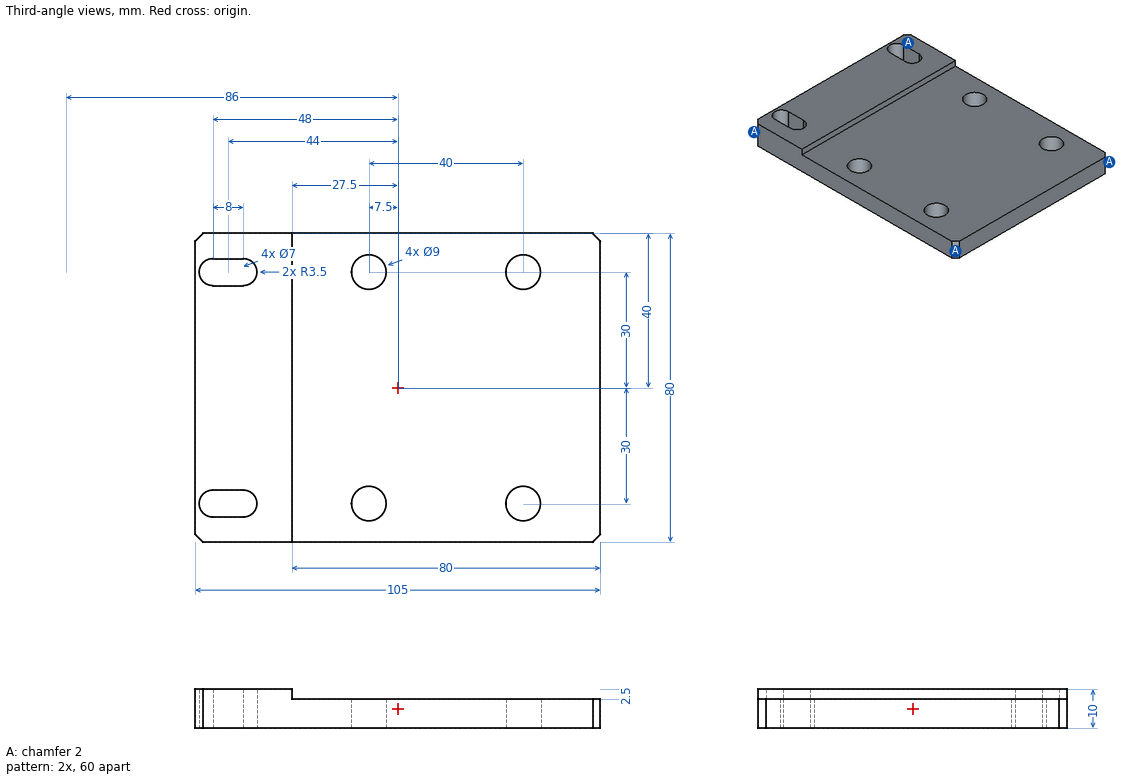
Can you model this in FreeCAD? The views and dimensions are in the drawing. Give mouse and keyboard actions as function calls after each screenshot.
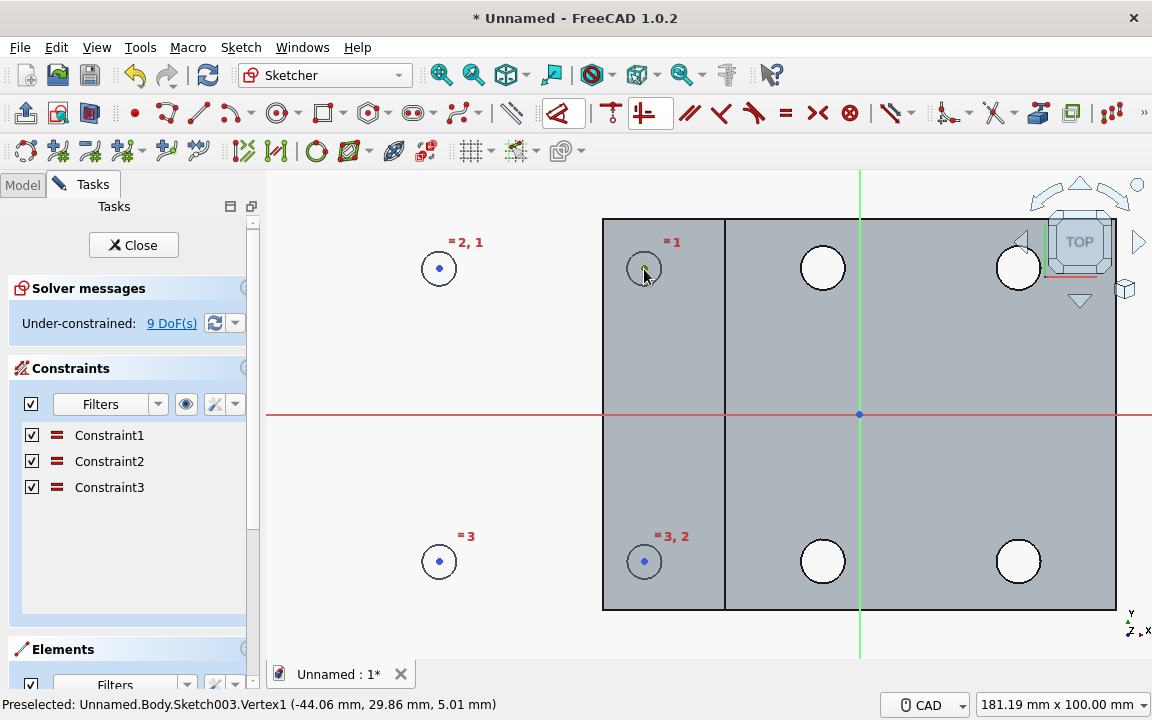
click(439, 269)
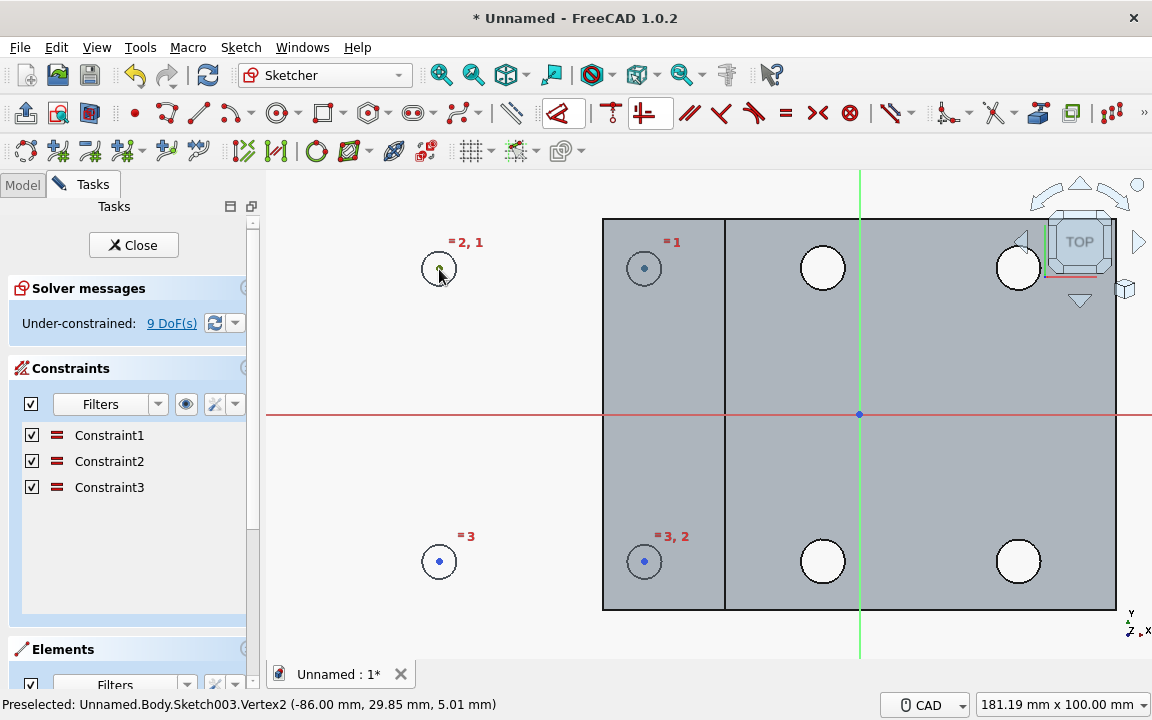
key(h)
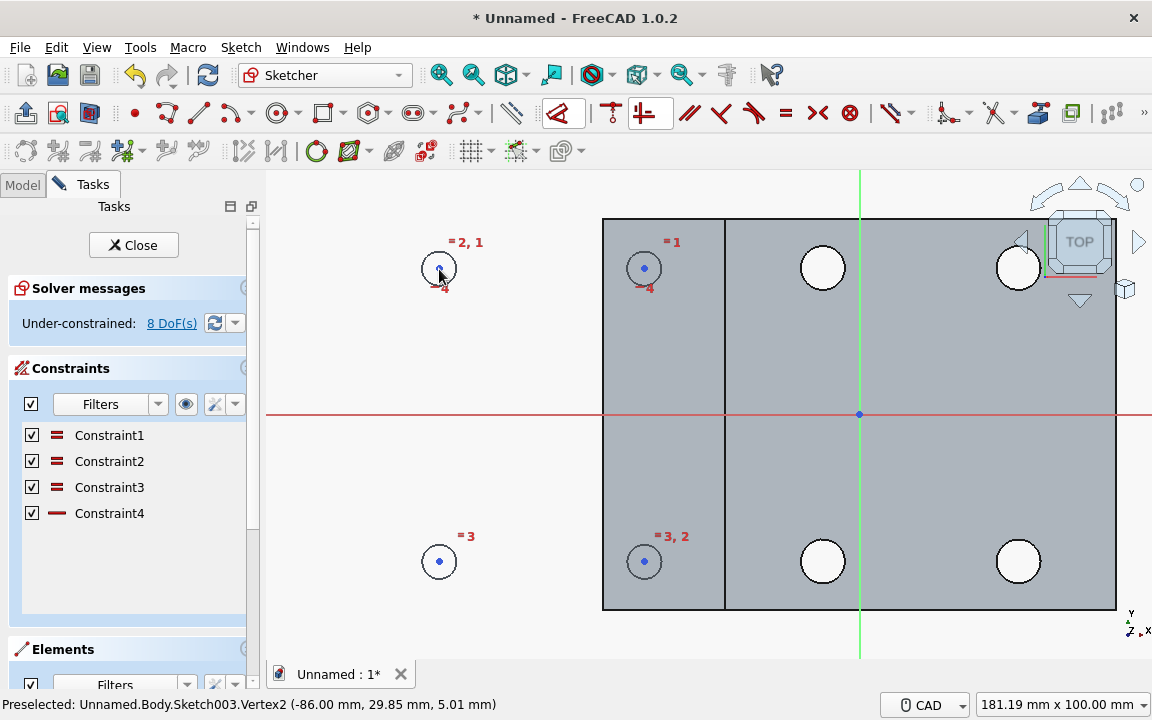
click(644, 269)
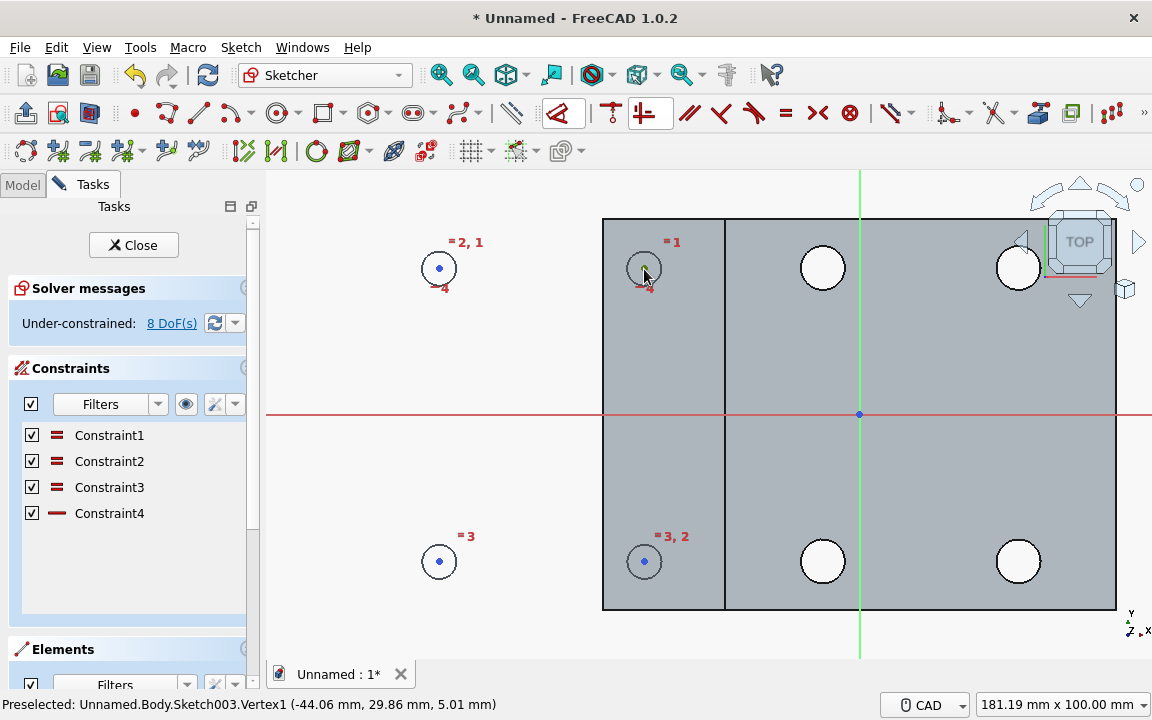
click(644, 562)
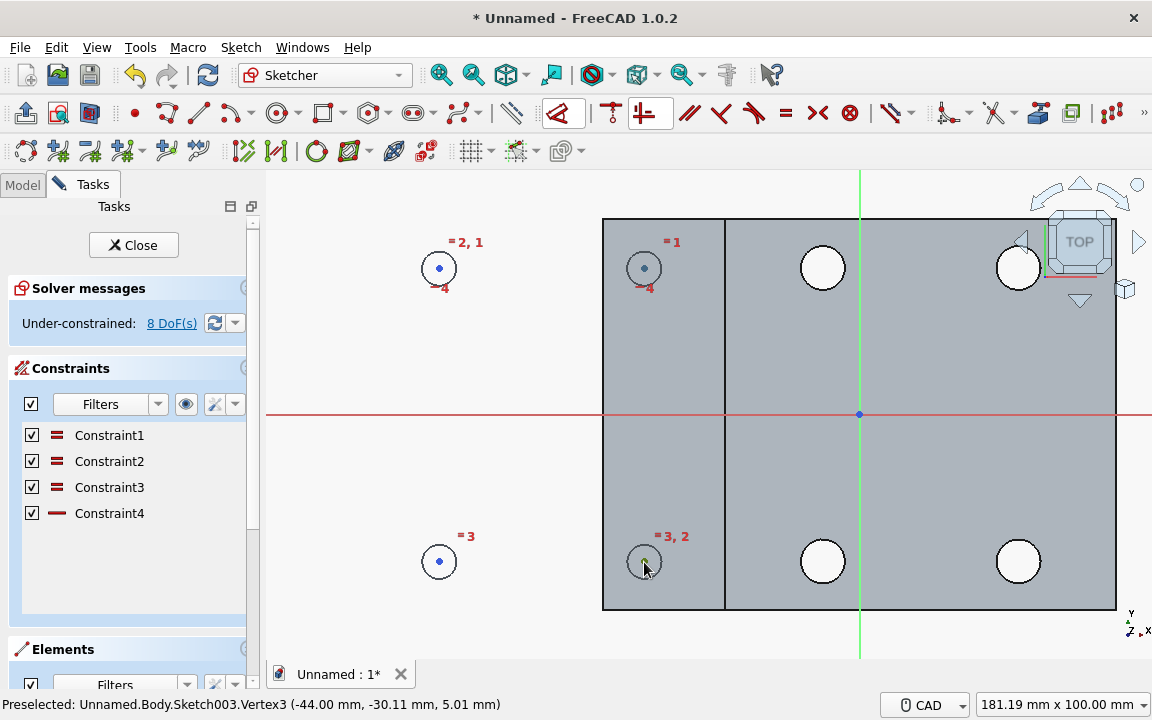
key(v)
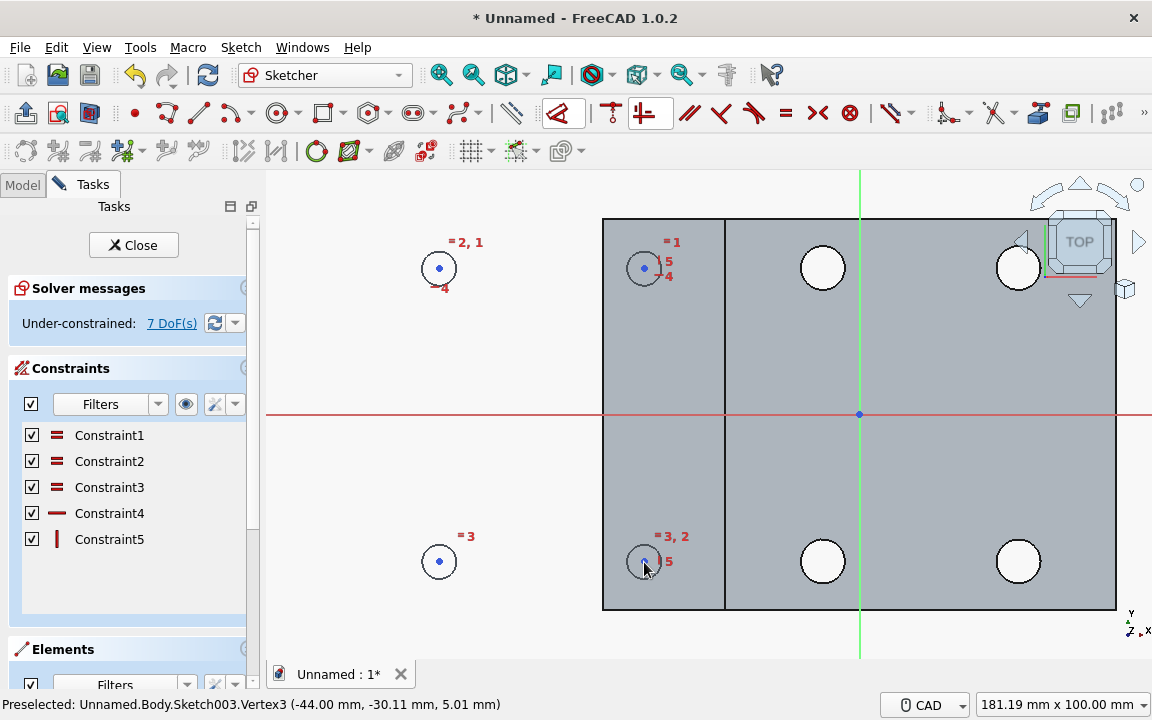
click(439, 269)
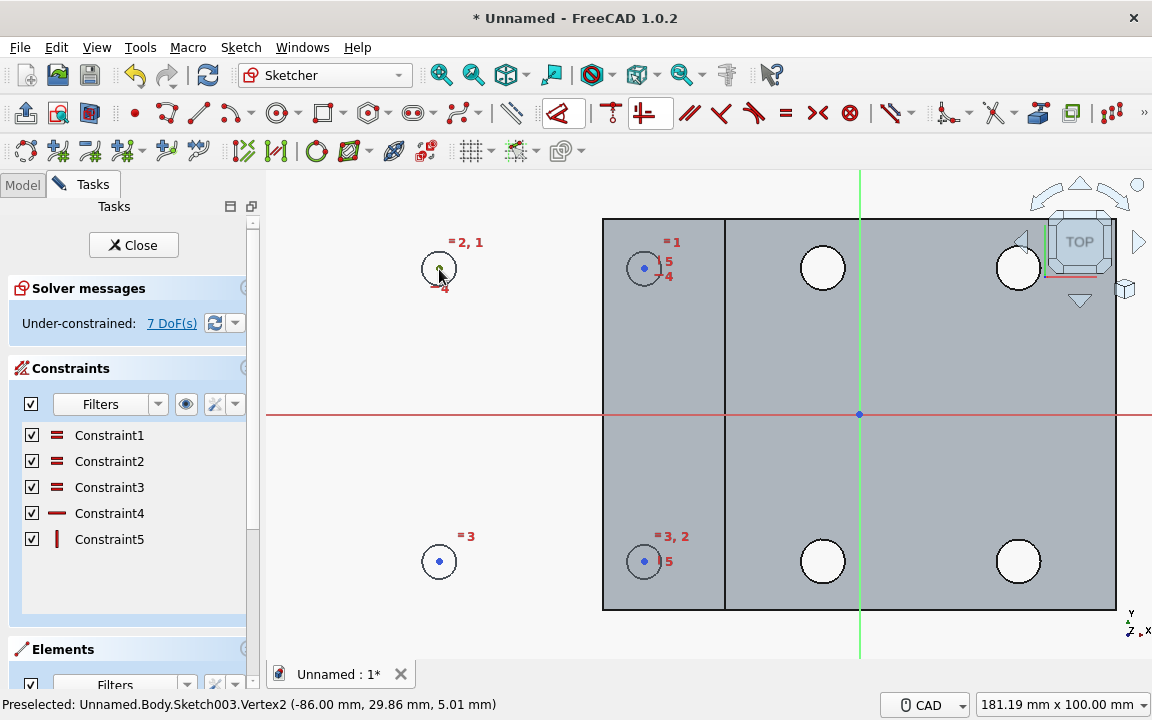
click(439, 562)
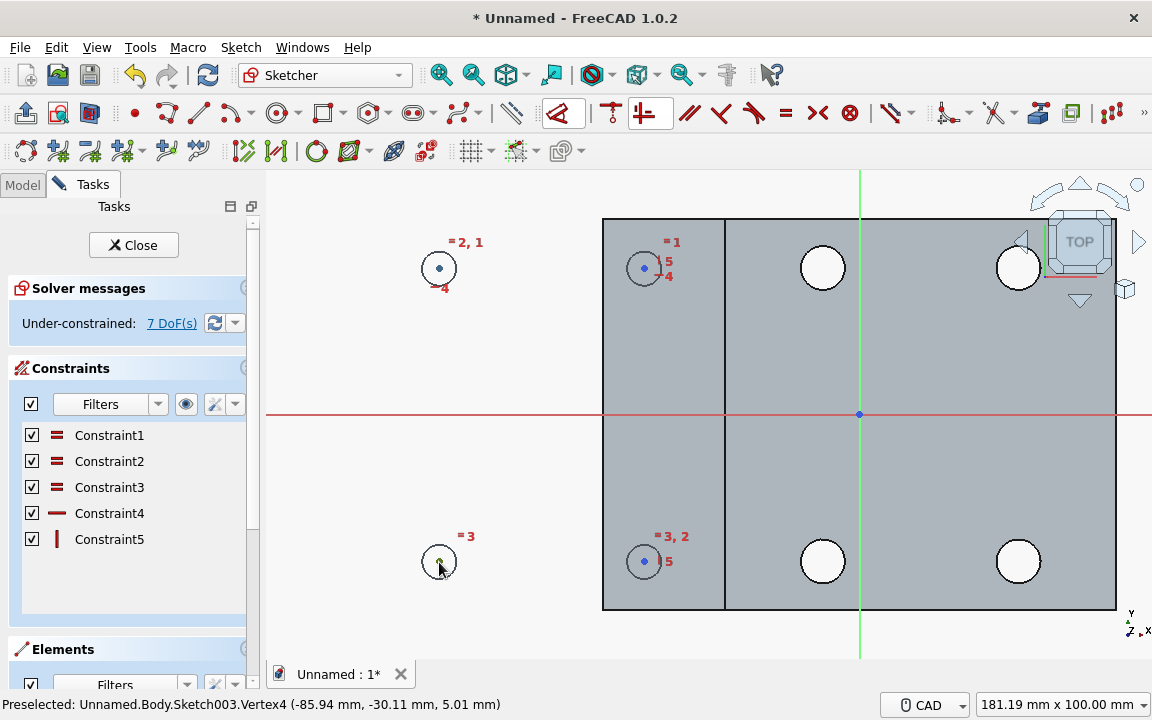
click(668, 114)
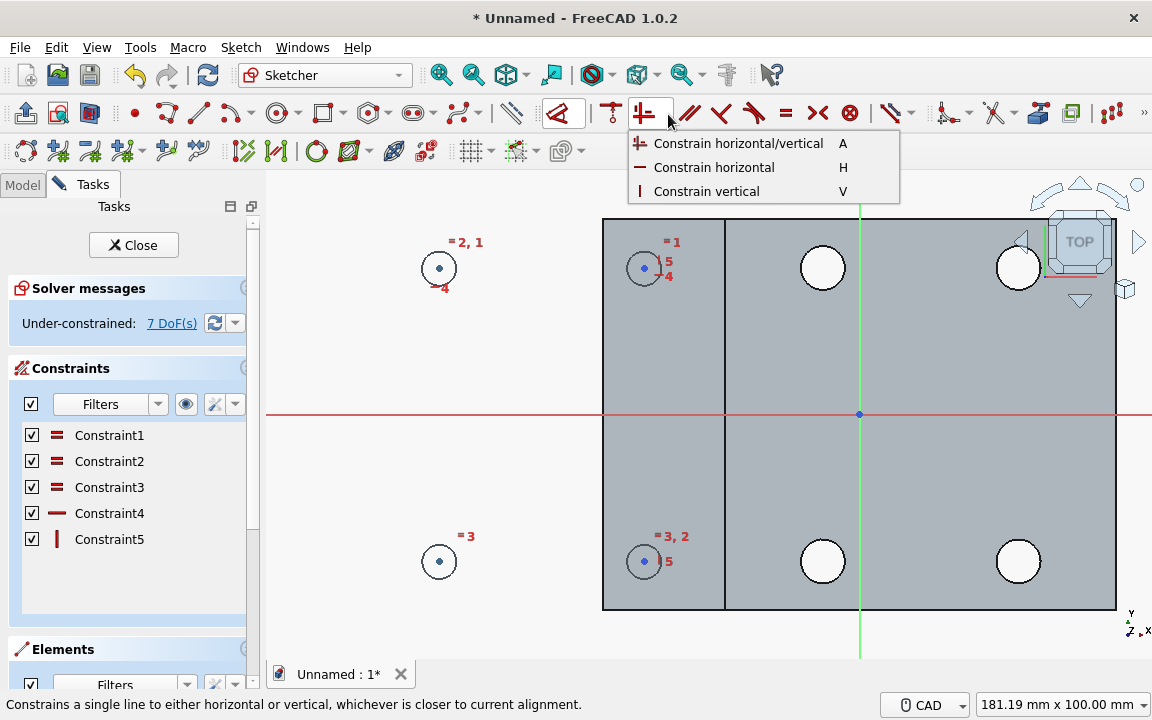
click(764, 191)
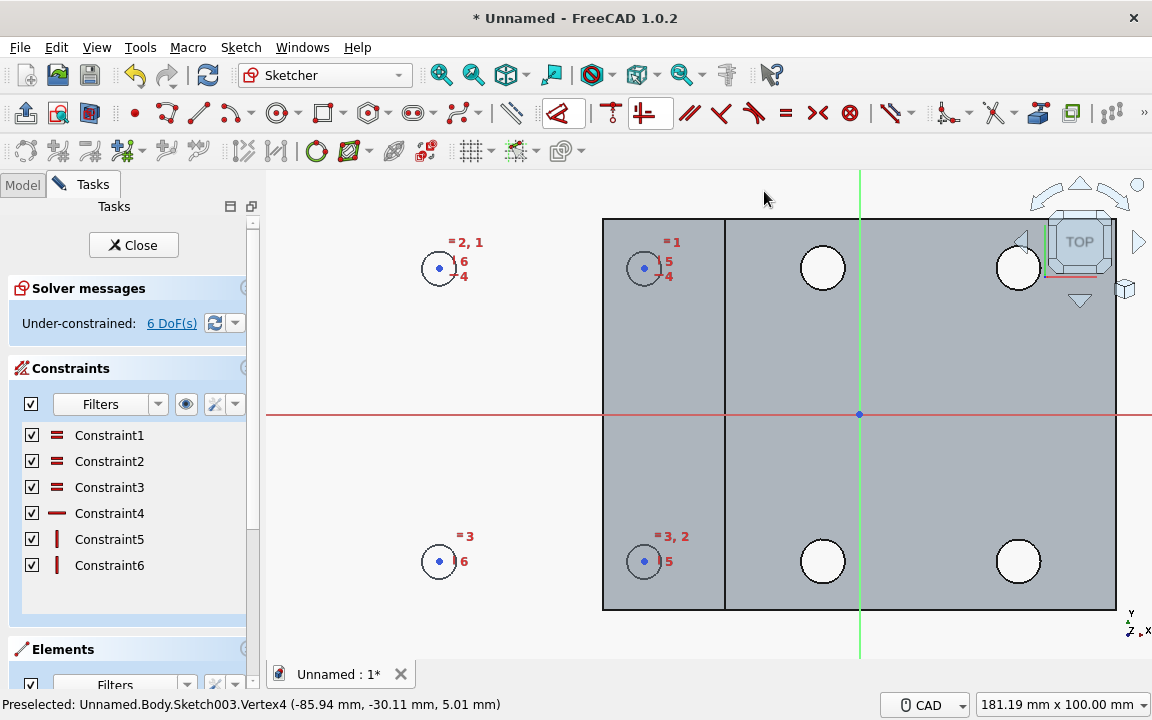
click(644, 562)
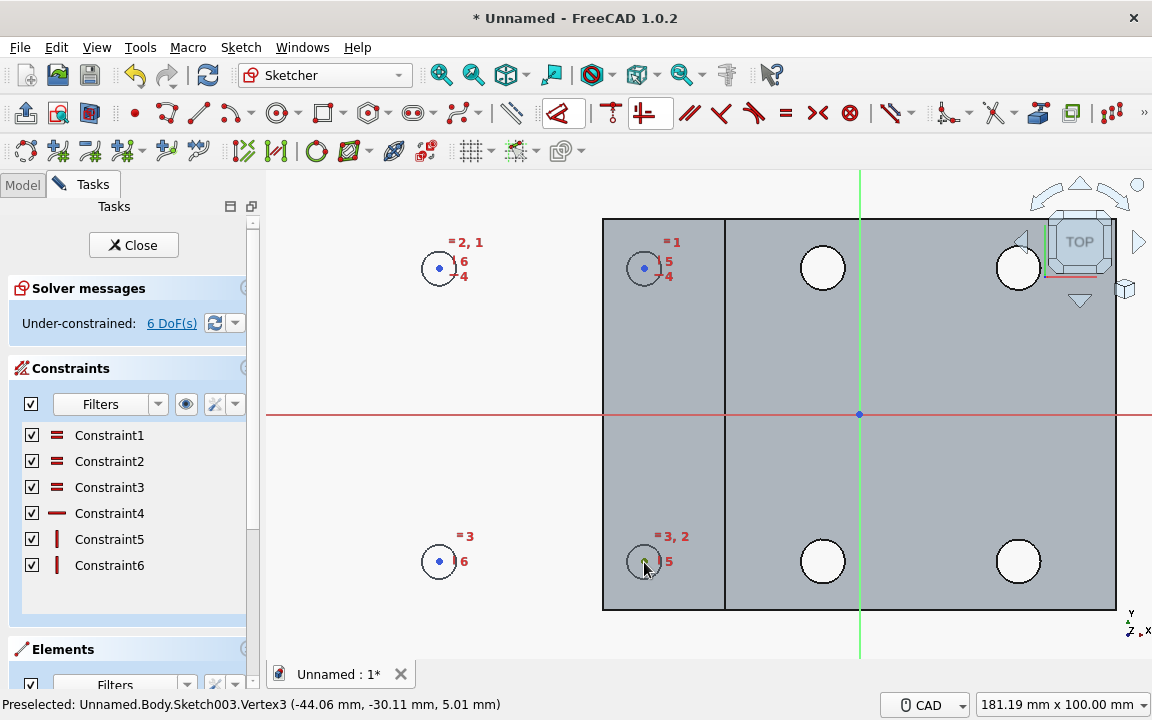
click(439, 562)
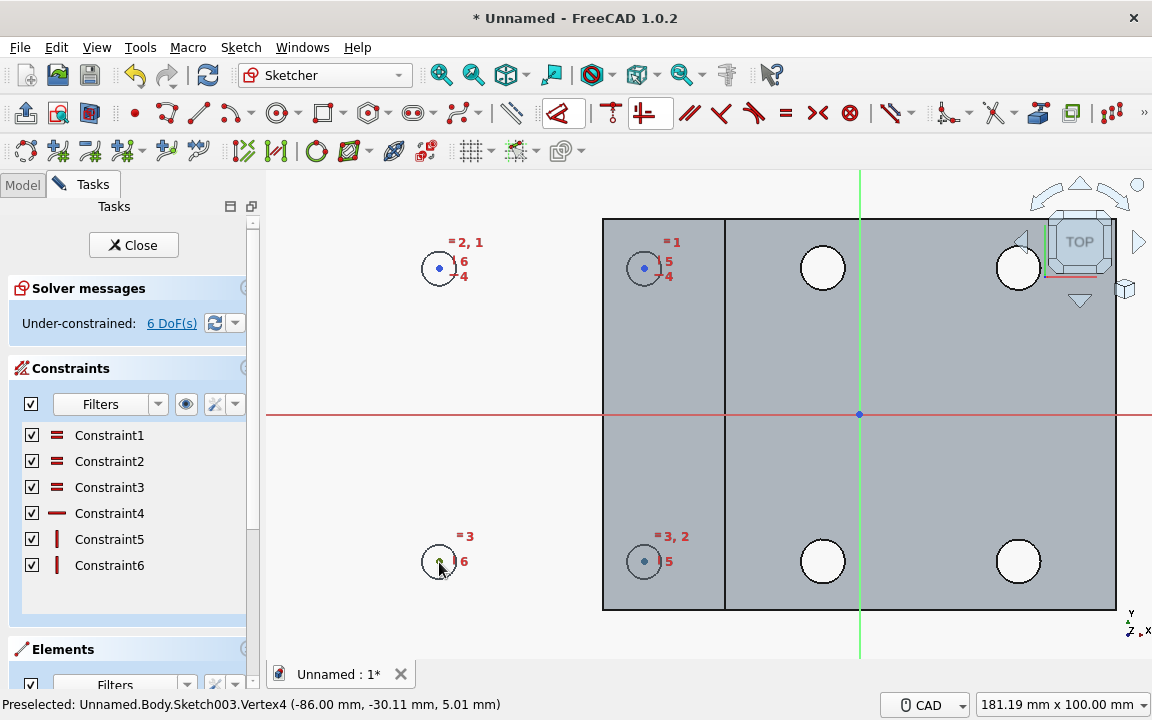
key(h)